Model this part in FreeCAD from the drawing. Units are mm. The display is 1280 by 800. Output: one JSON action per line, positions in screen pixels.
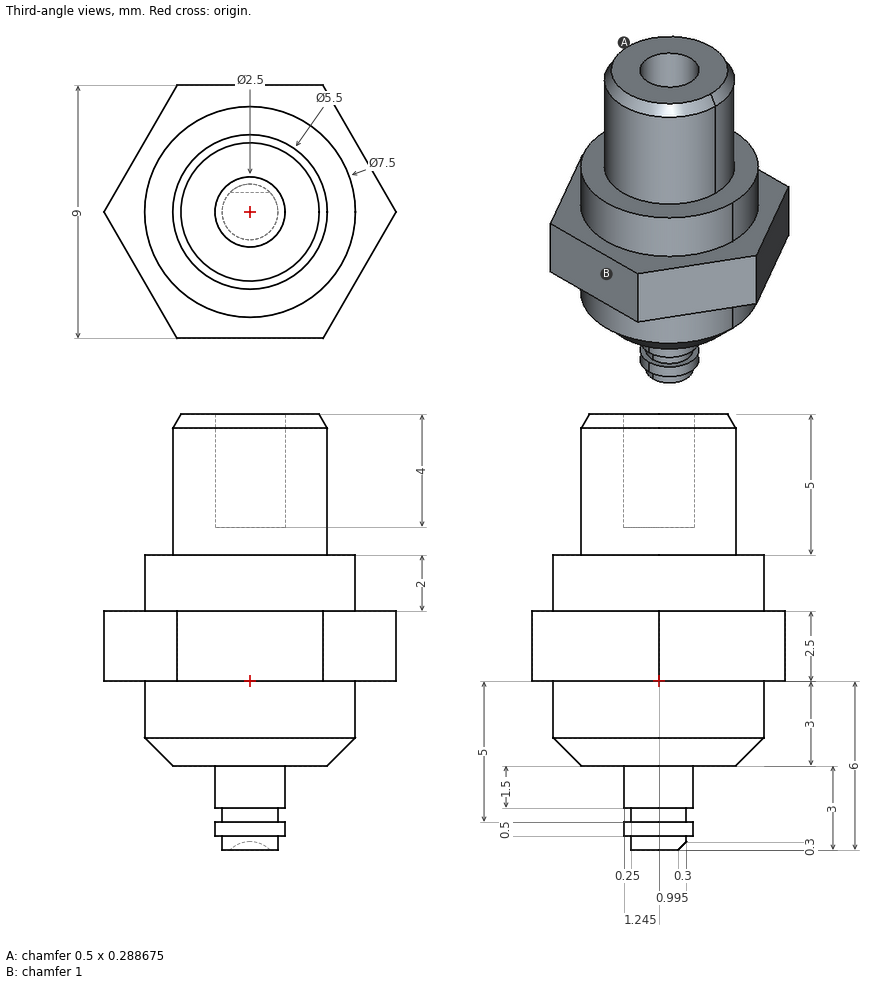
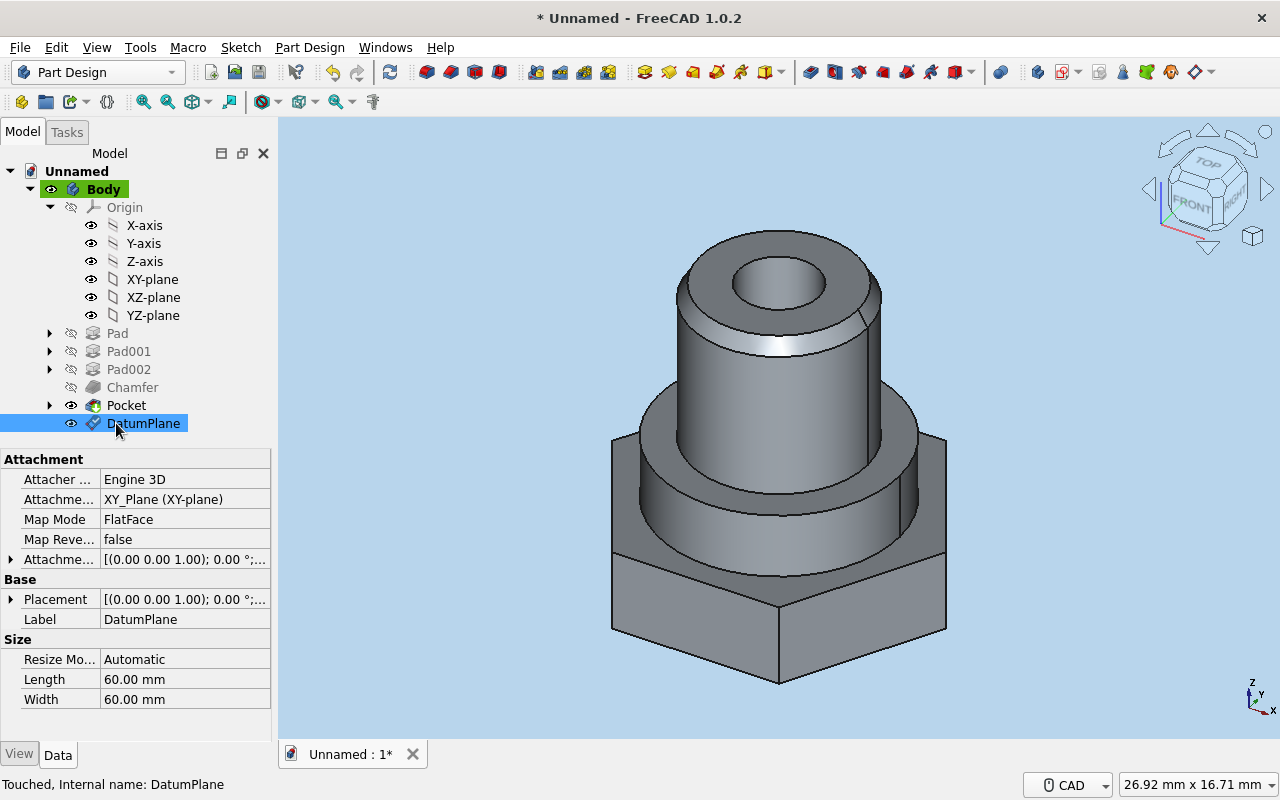
{"action": "left_click", "coordinate": [1062, 72]}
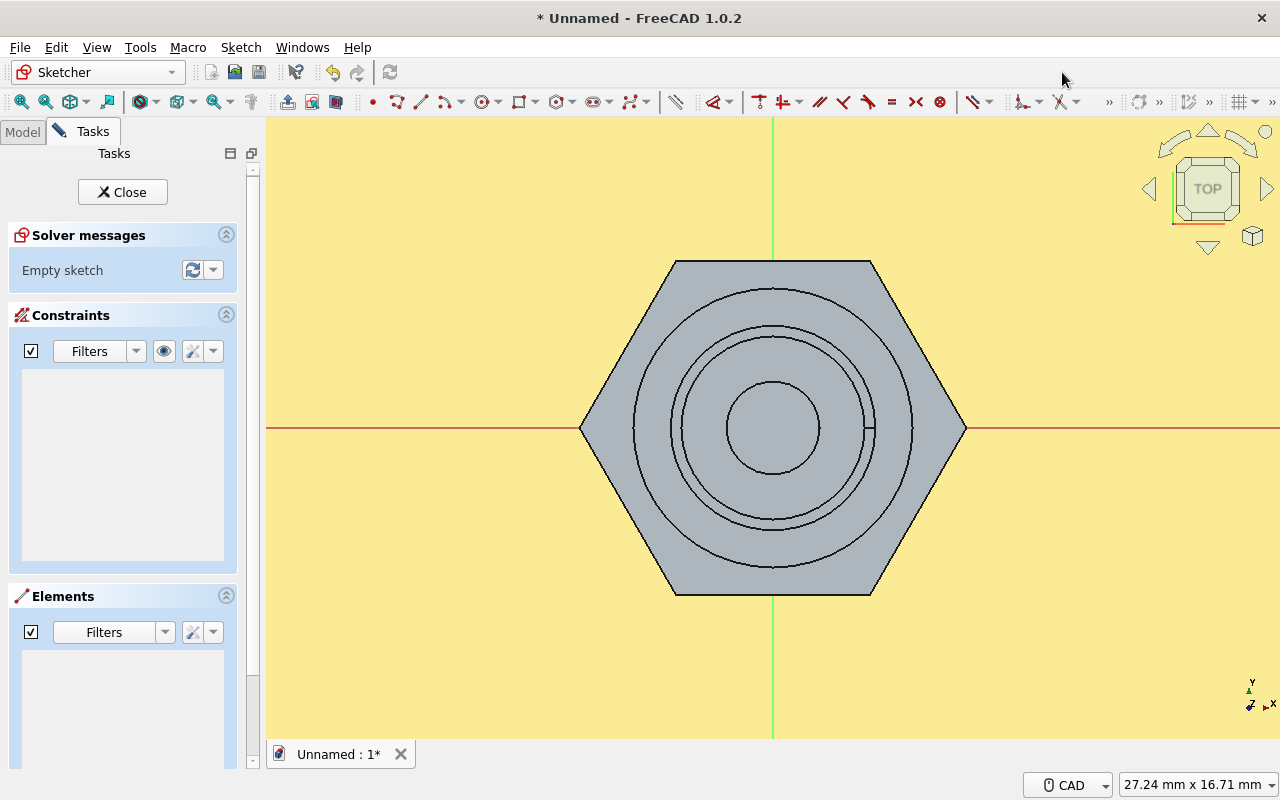
{"action": "key", "text": "q s"}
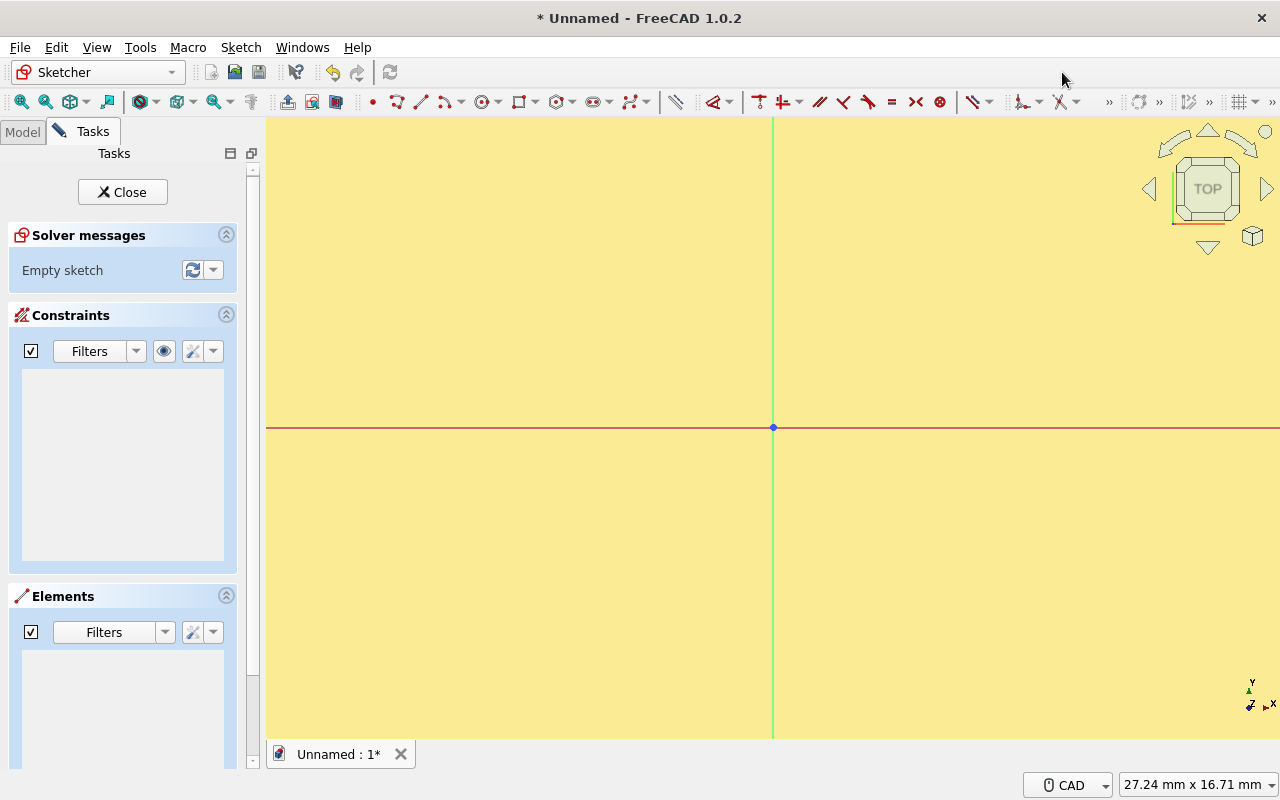
{"action": "scroll", "coordinate": [912, 428], "scroll_direction": "up", "scroll_amount": 2}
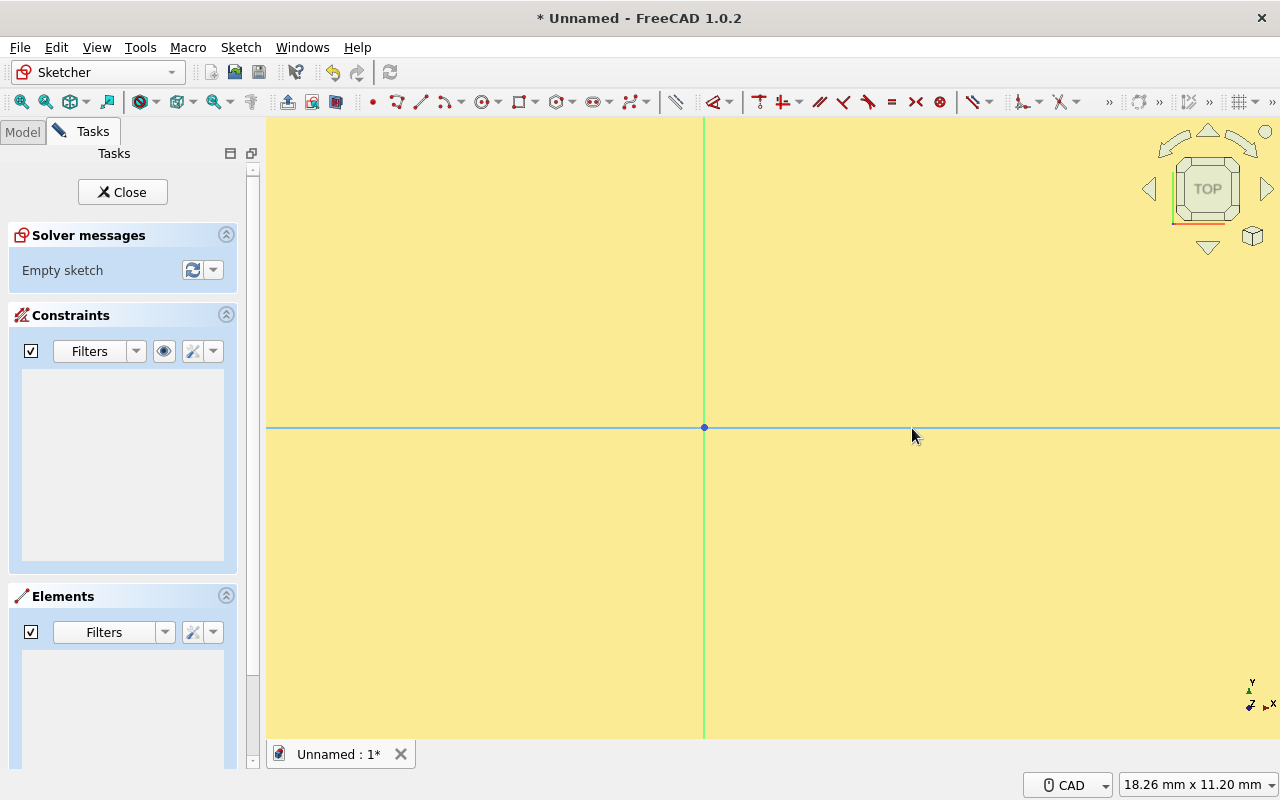
{"action": "key", "text": "g c"}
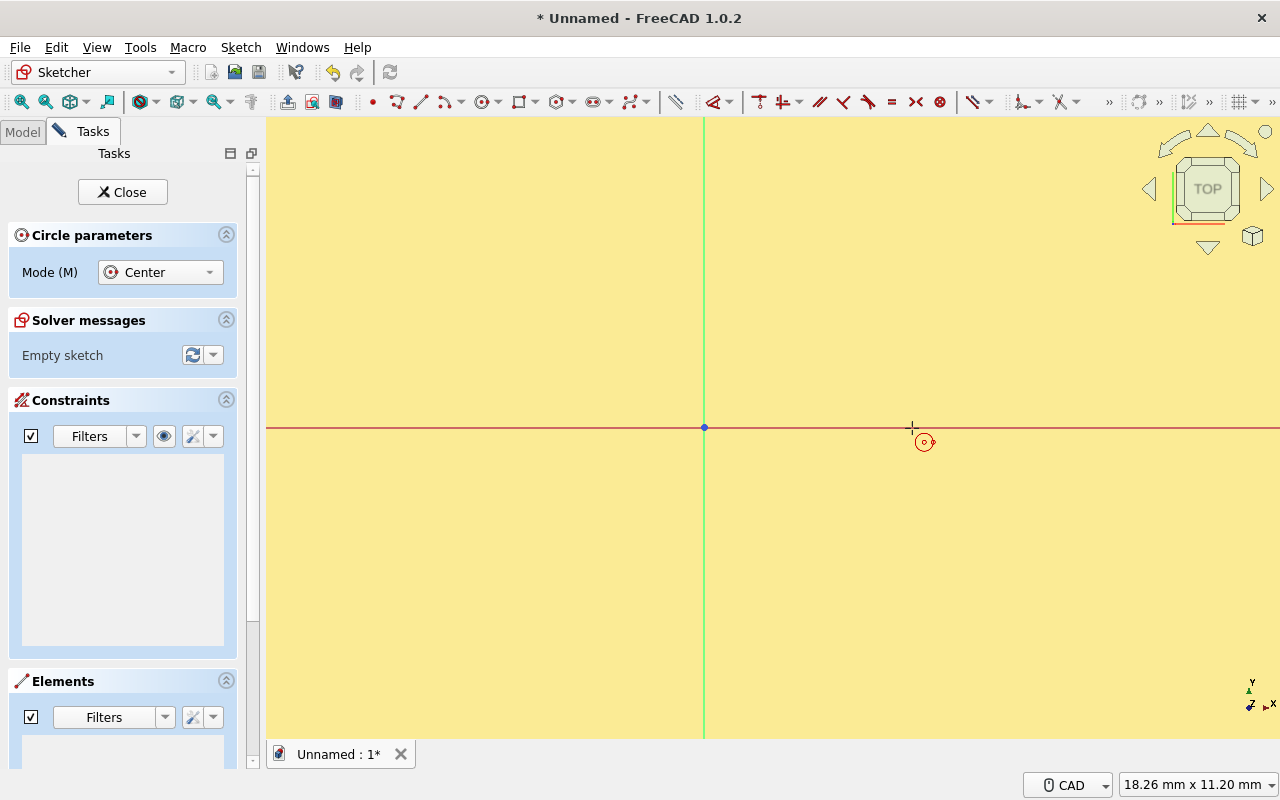
{"action": "left_click", "coordinate": [704, 428]}
{"action": "left_click", "coordinate": [852, 281]}
{"action": "key", "text": "Escape"}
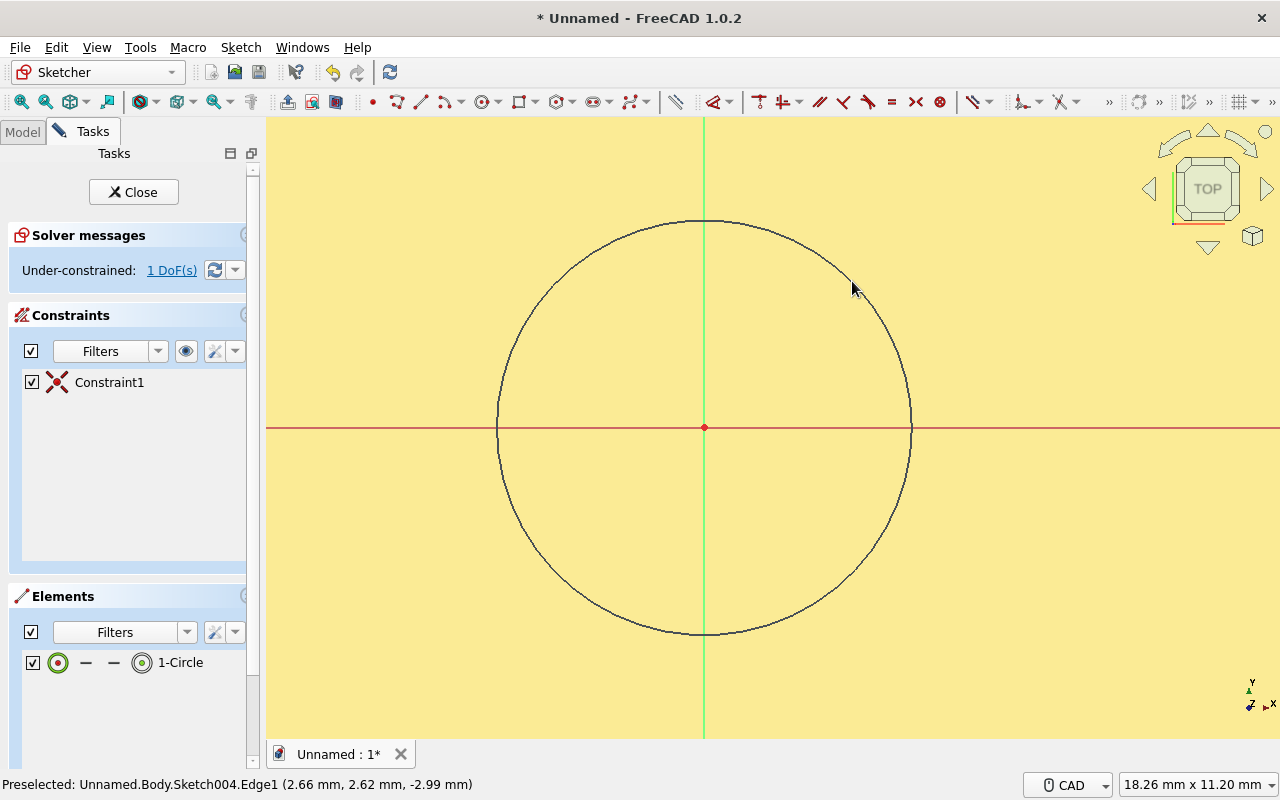
{"action": "left_click", "coordinate": [851, 281]}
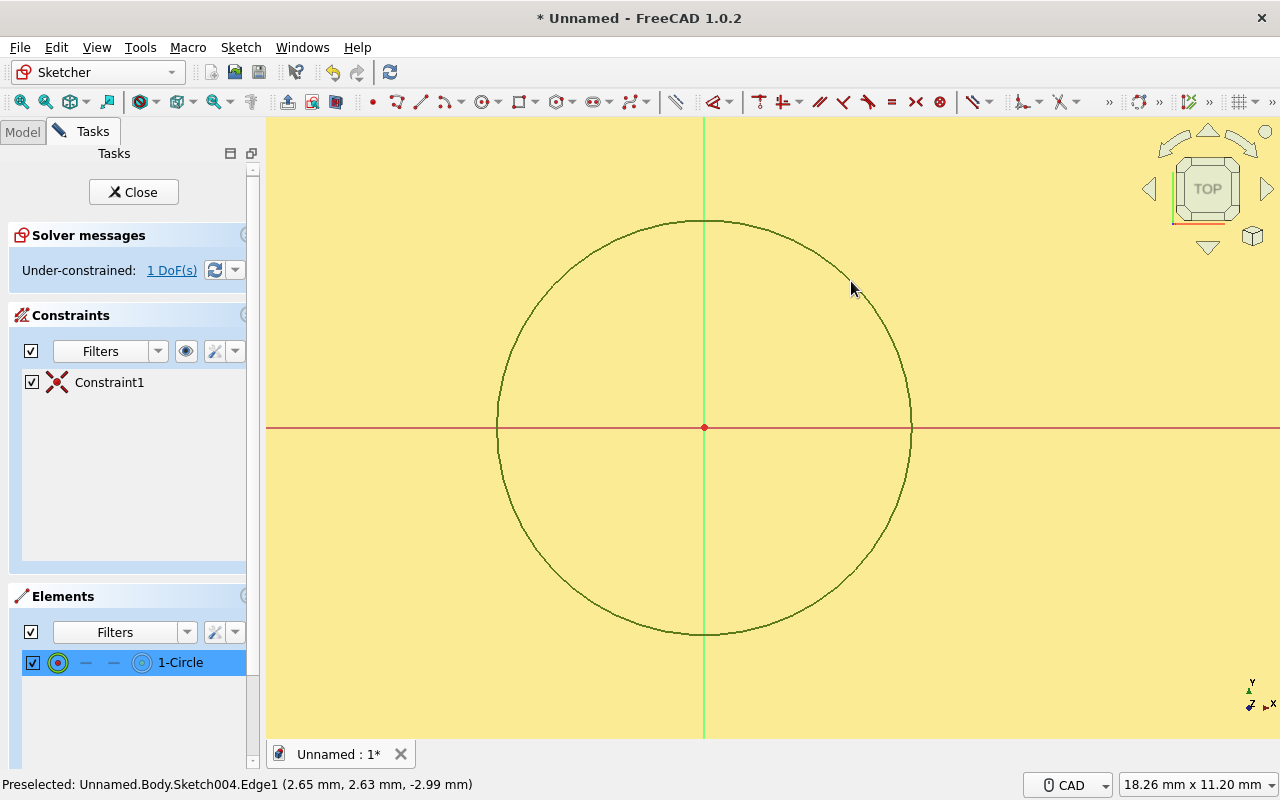
{"action": "key", "text": "k o"}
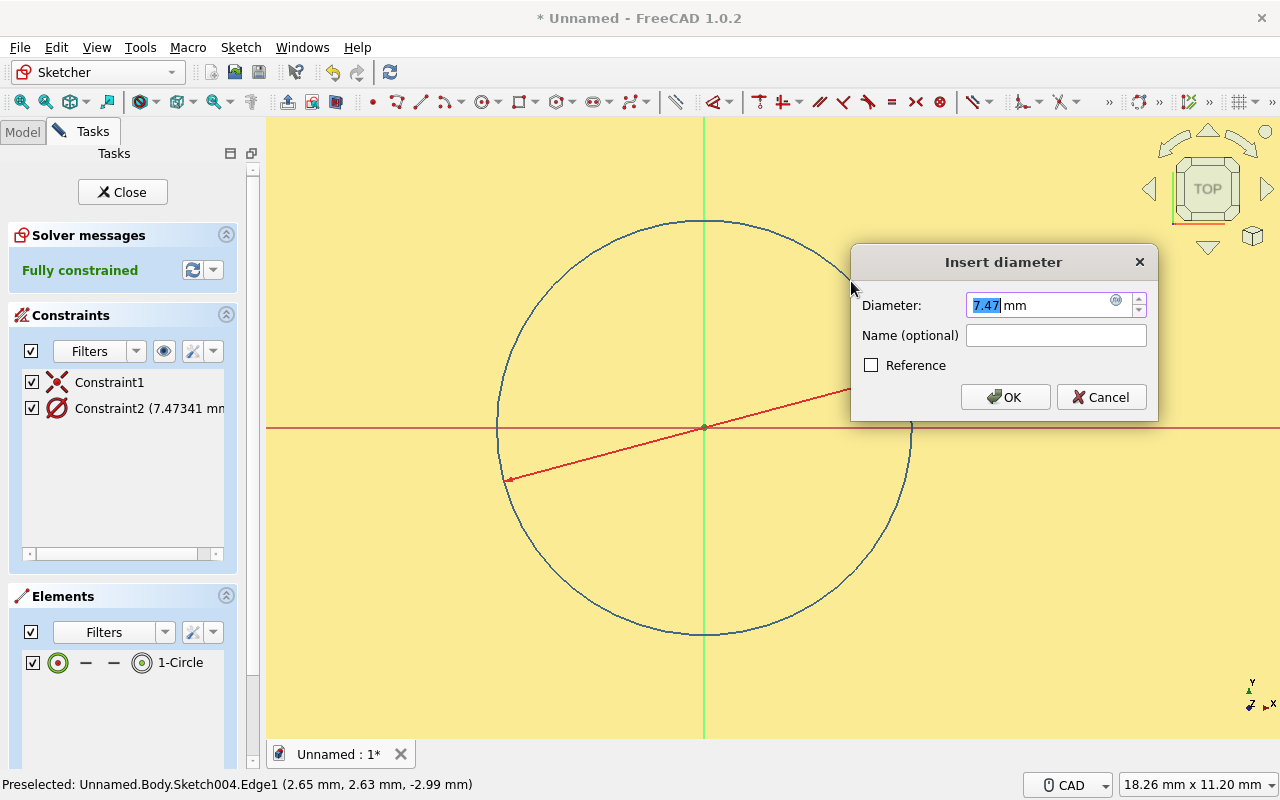
{"action": "type", "text": "7.5"}
{"action": "key", "text": "Return"}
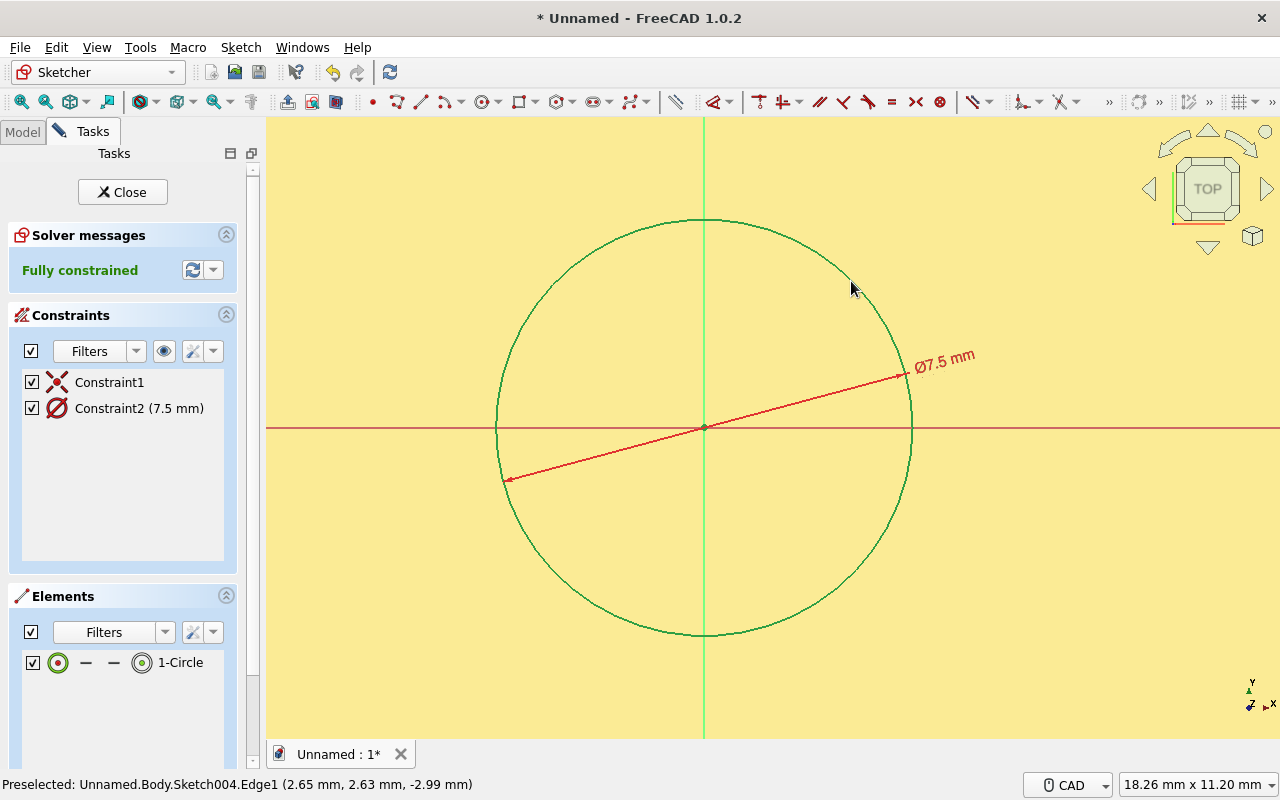
{"action": "left_click", "coordinate": [123, 192]}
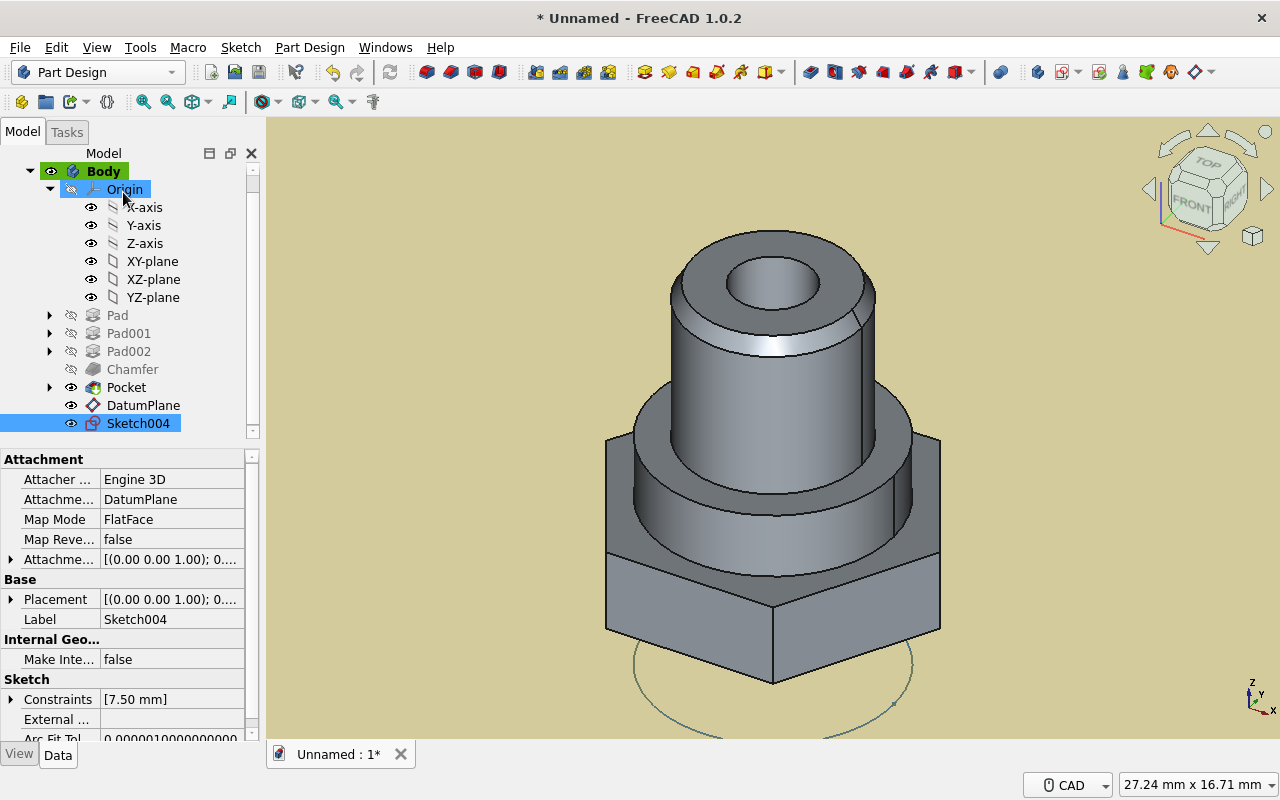
{"action": "left_click", "coordinate": [646, 72]}